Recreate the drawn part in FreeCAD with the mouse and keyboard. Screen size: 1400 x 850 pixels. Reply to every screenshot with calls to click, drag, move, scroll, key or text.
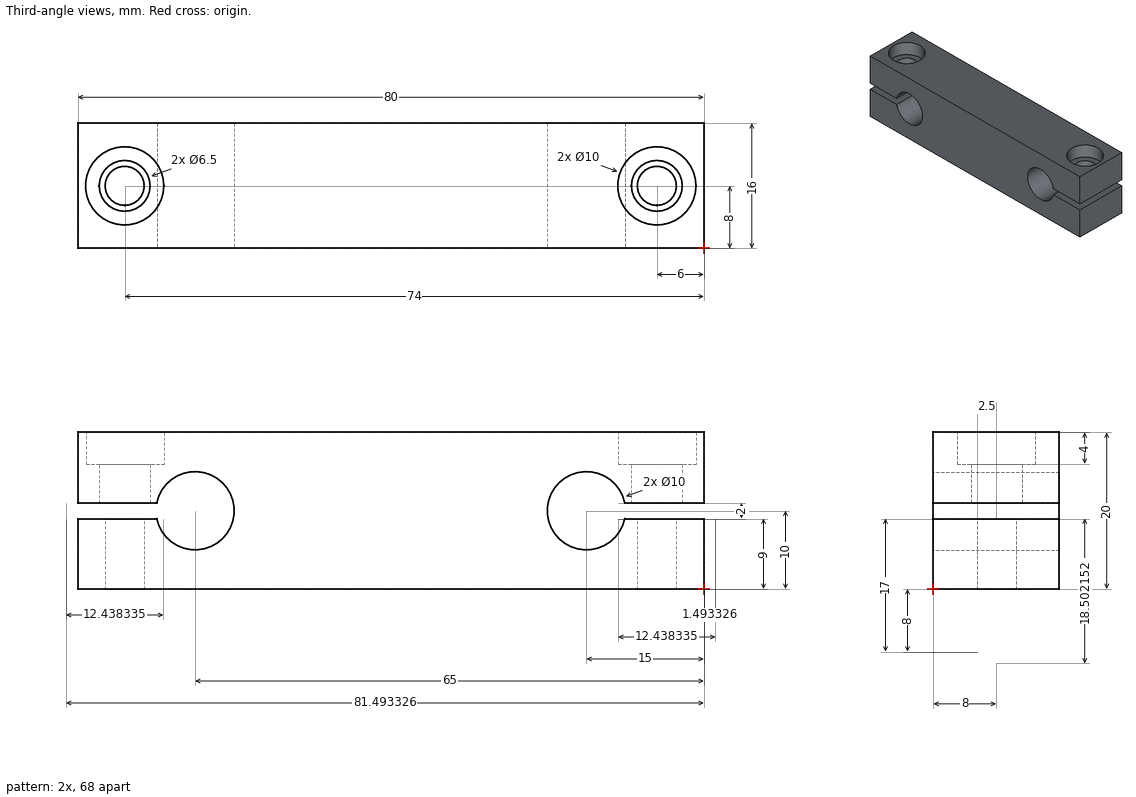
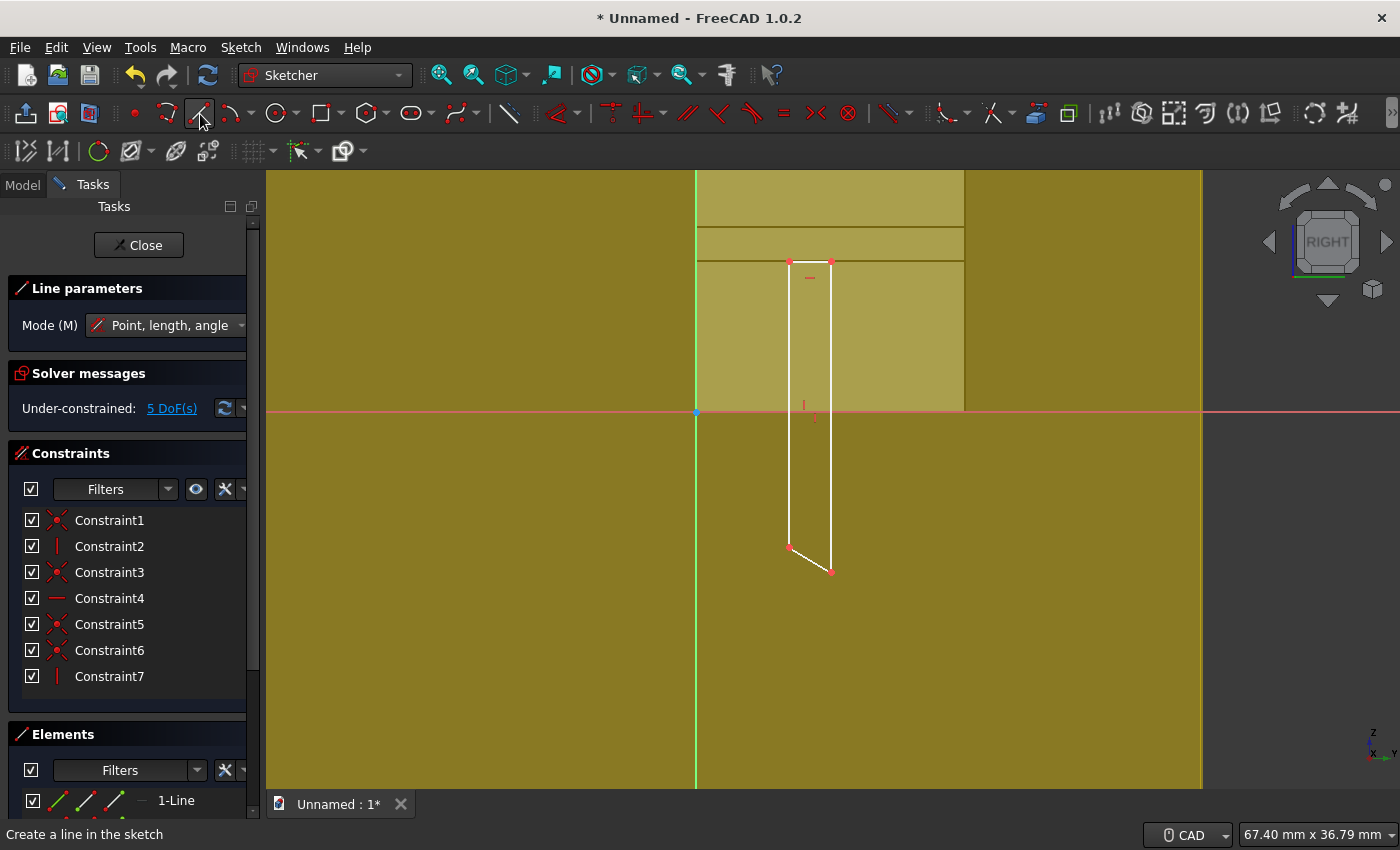
click(831, 603)
click(831, 697)
key(Escape)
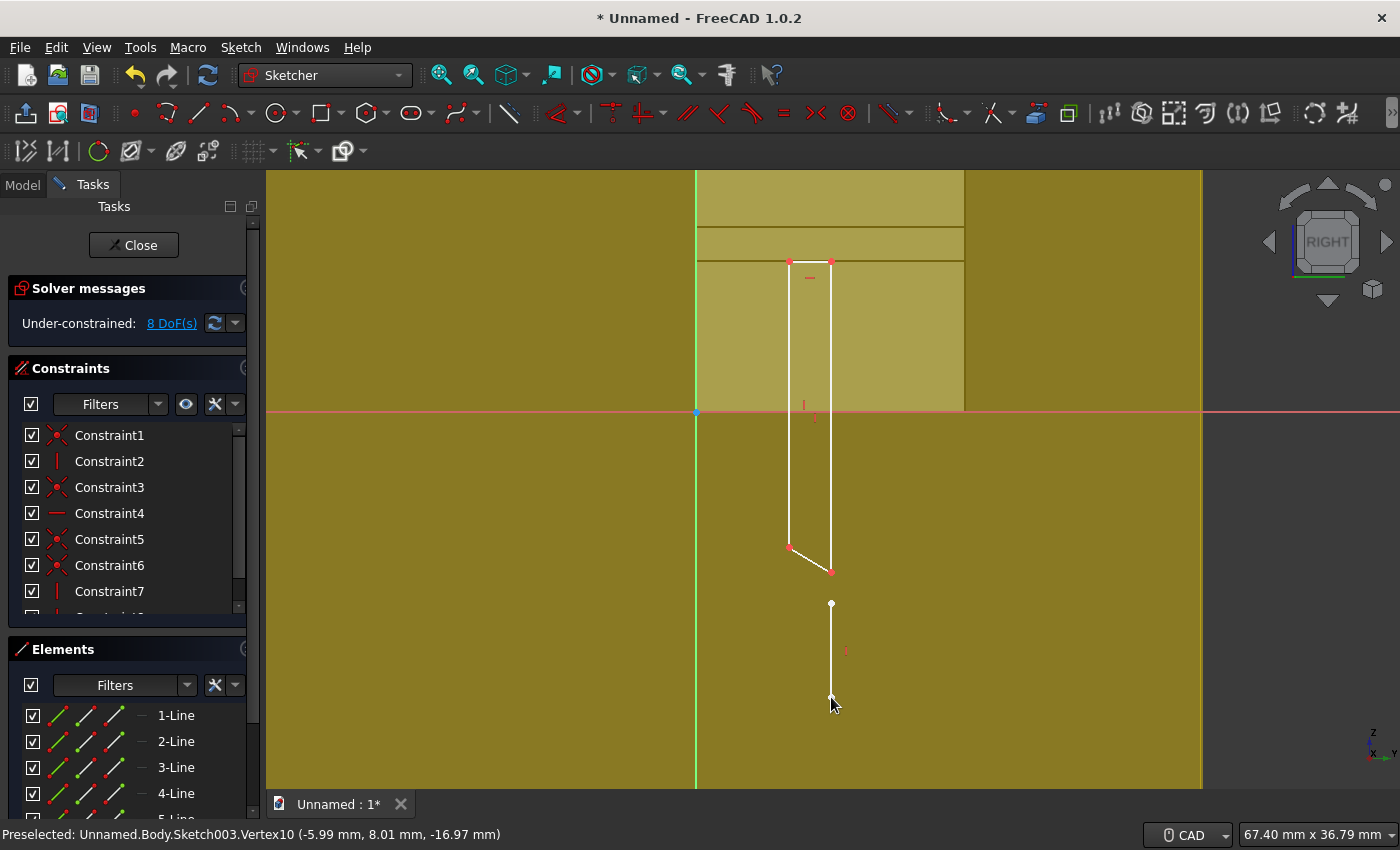
click(831, 632)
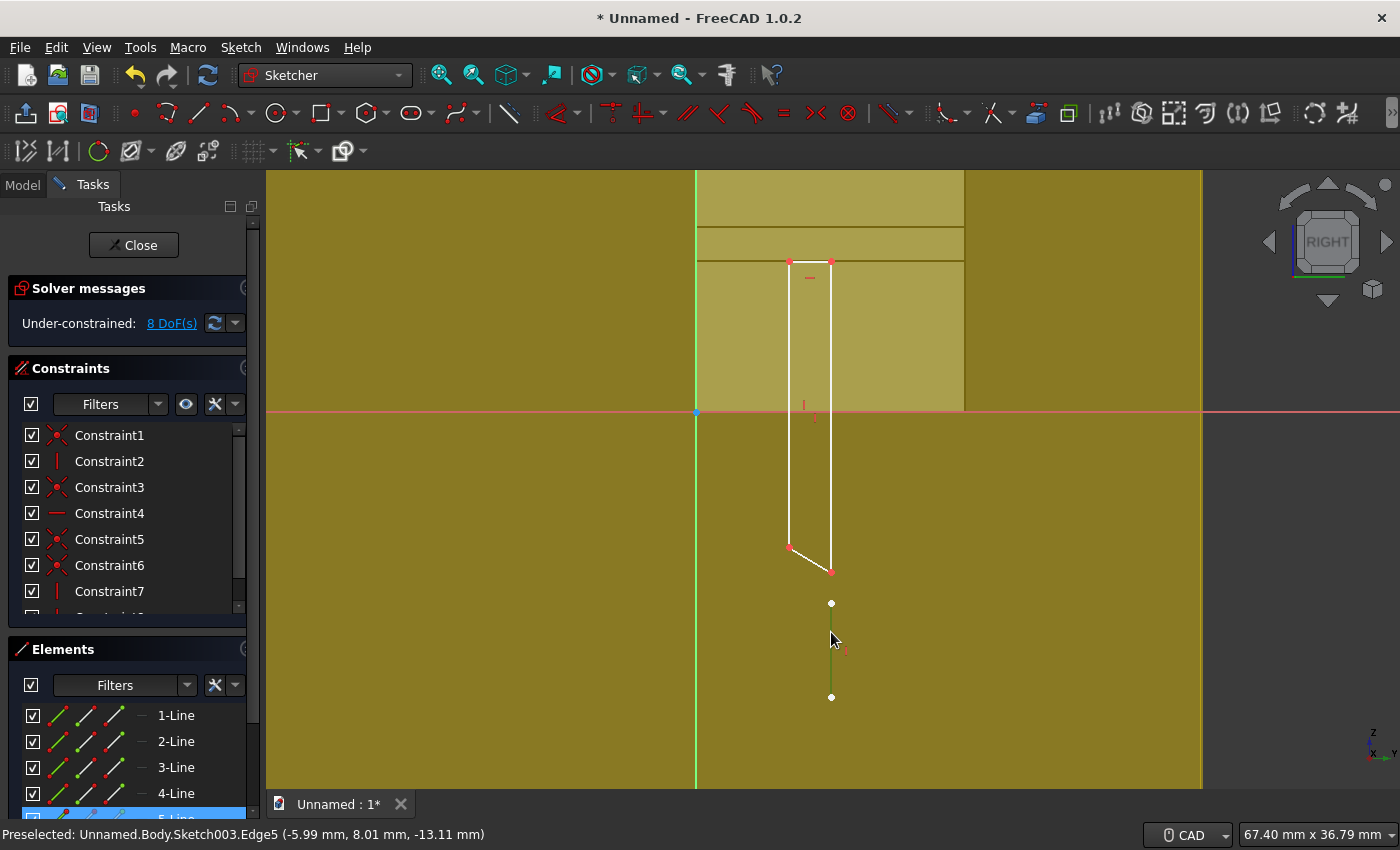
click(510, 114)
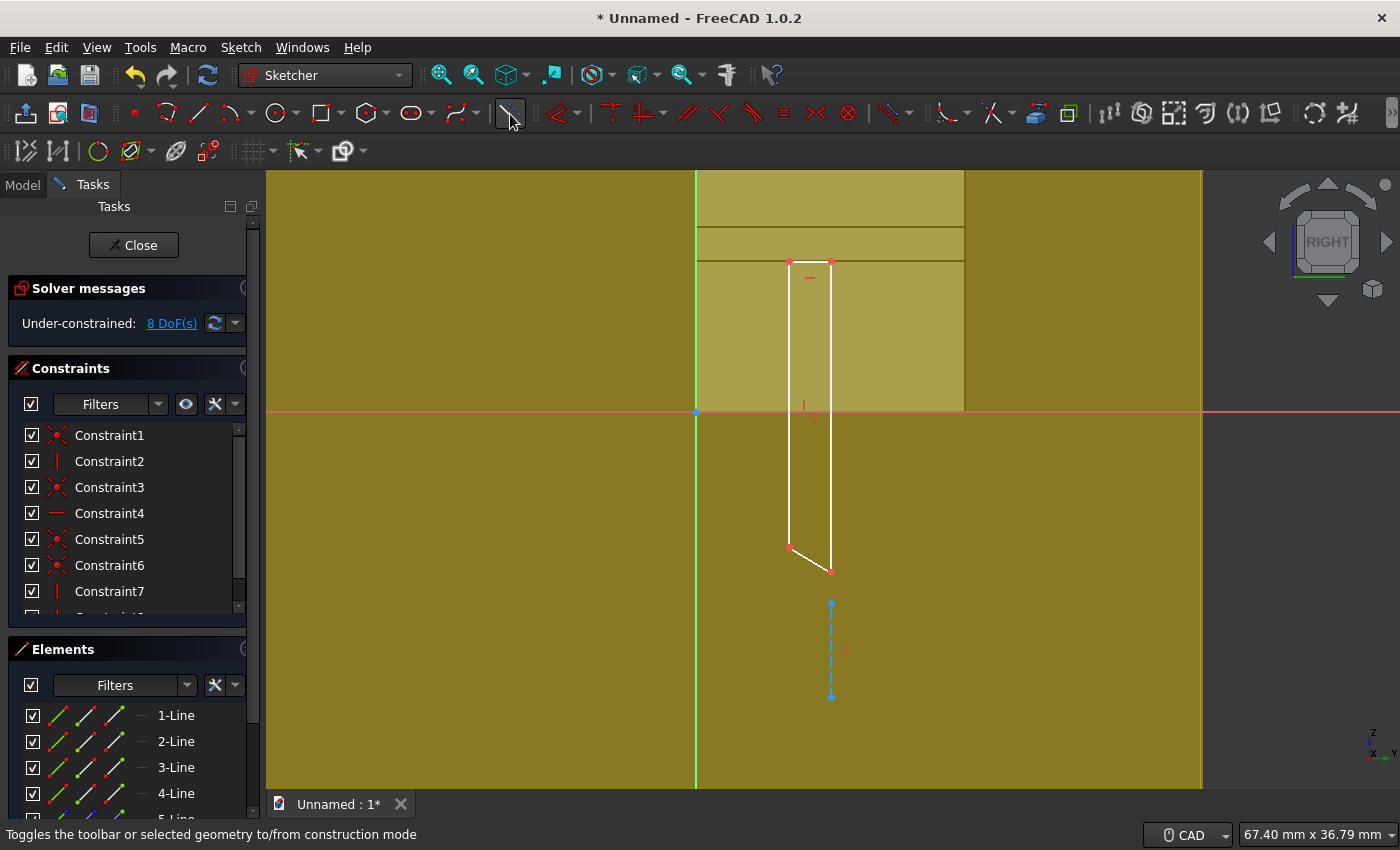
click(556, 114)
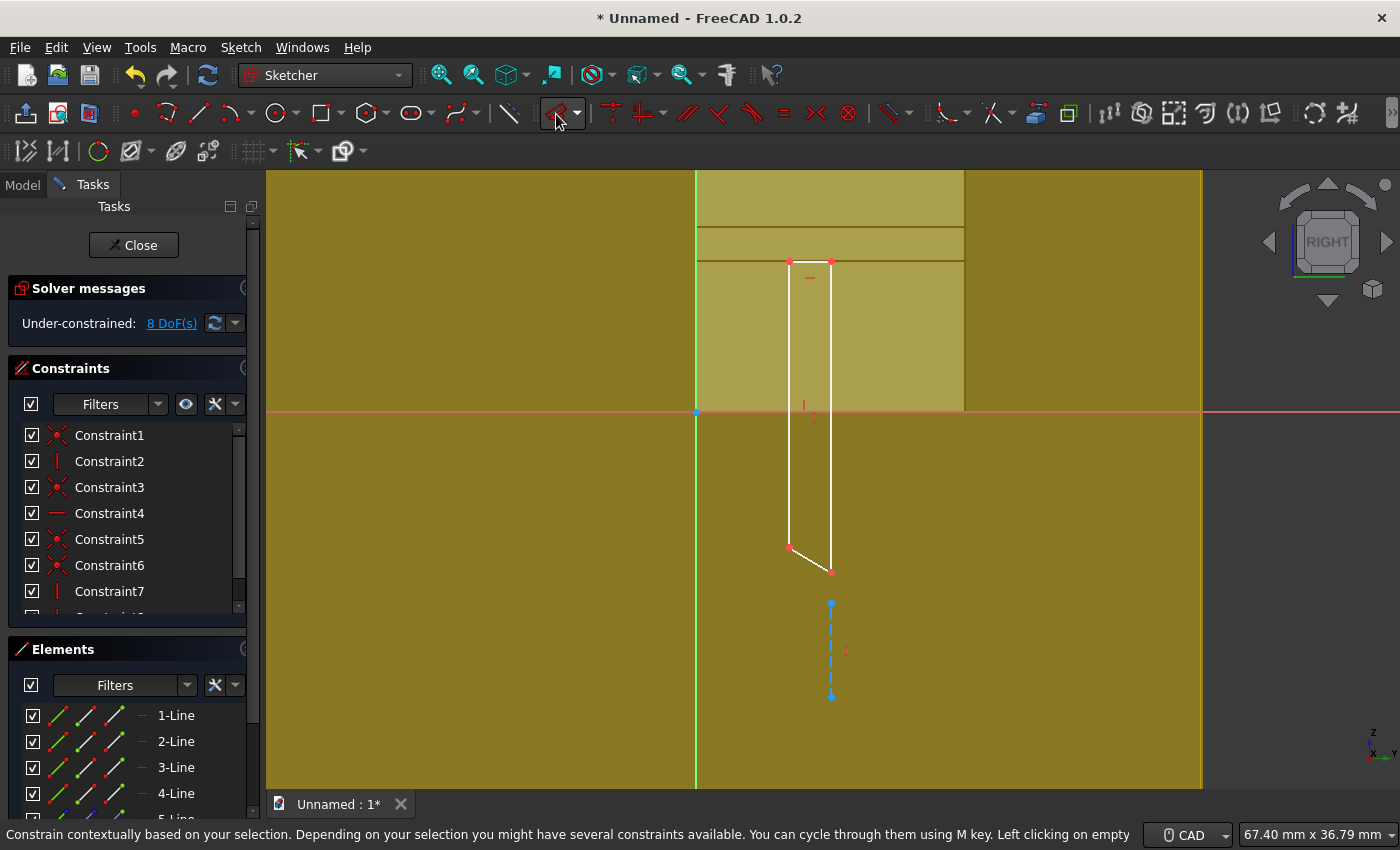
click(789, 348)
click(755, 339)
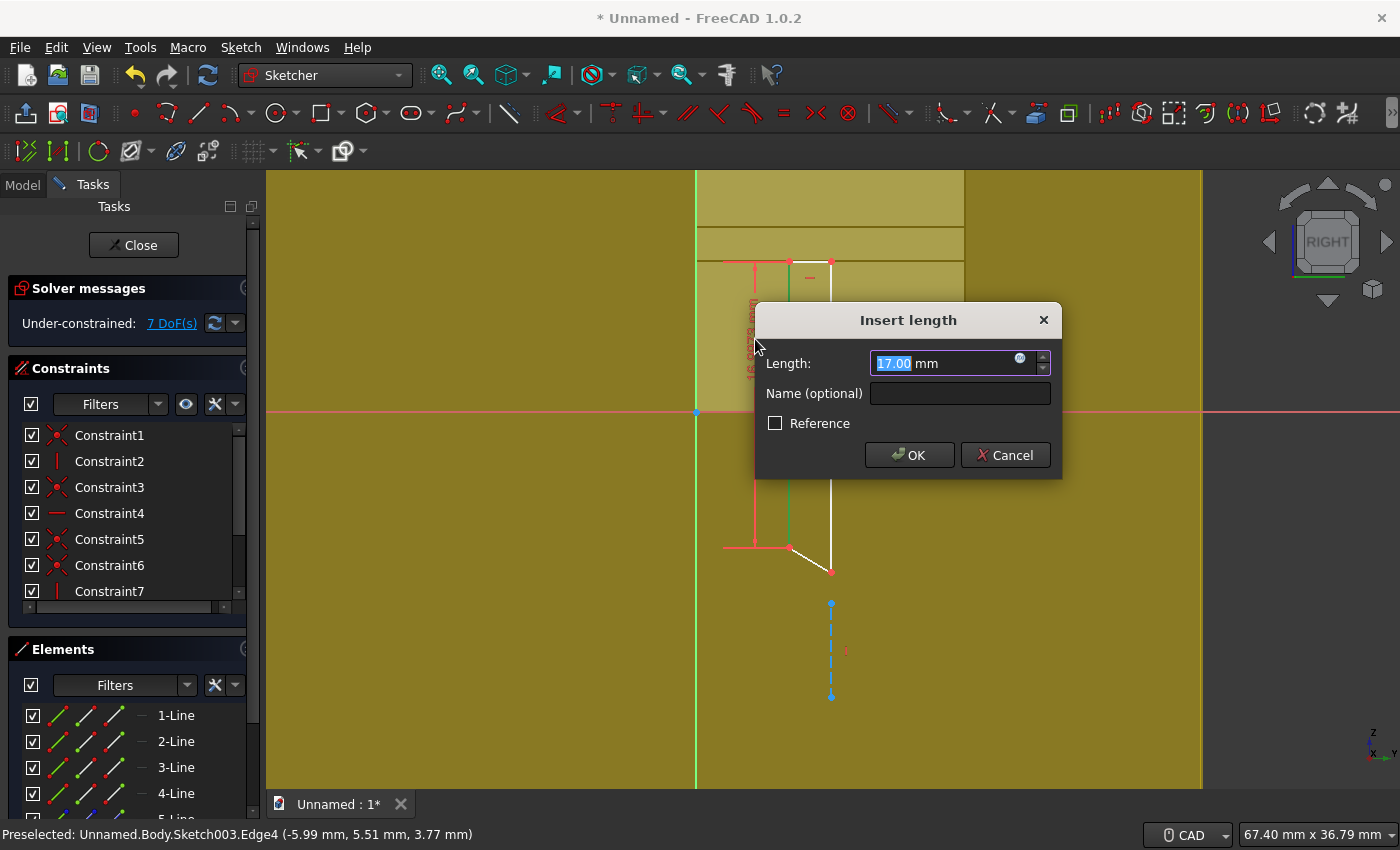
text(17)
key(Return)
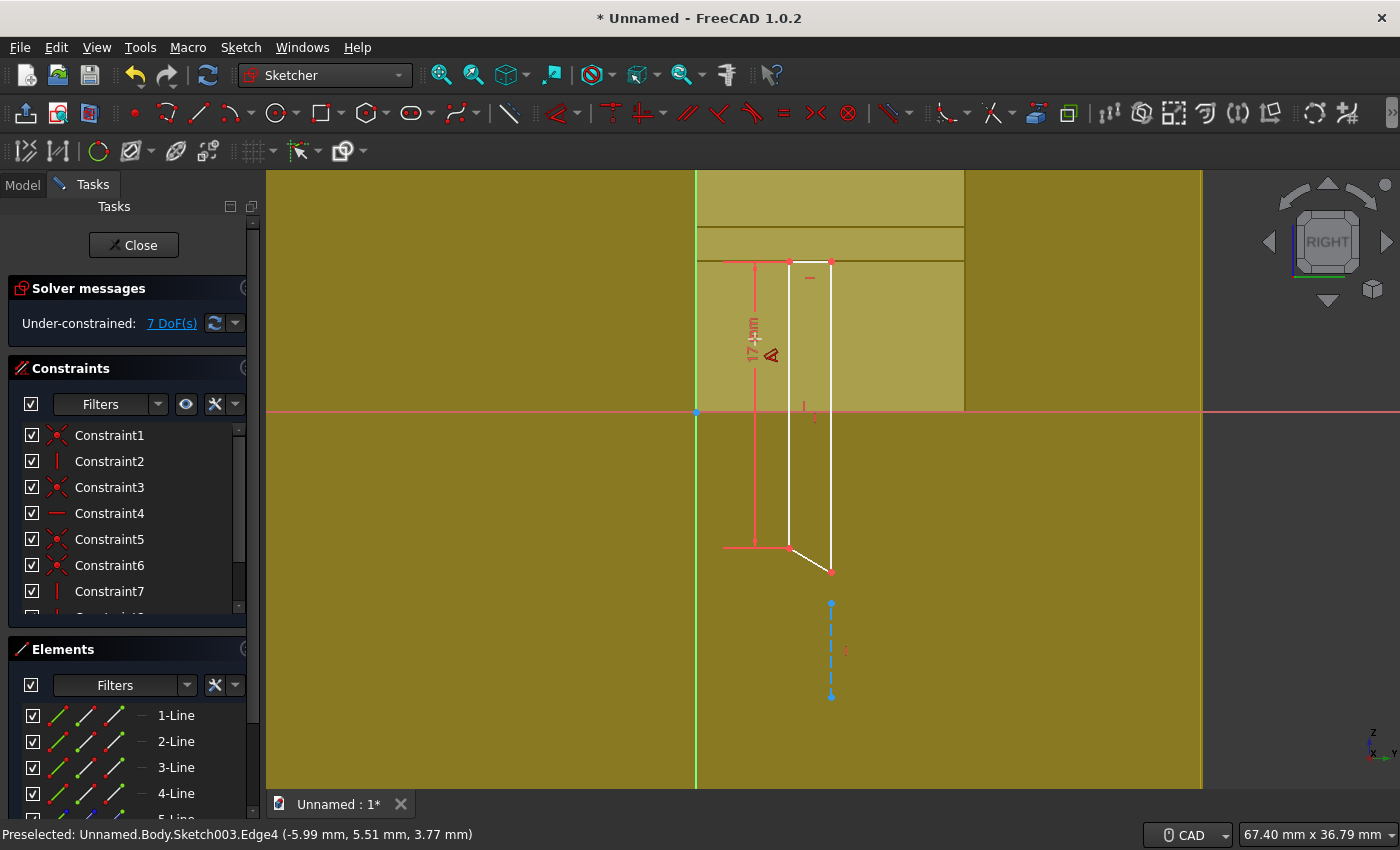
click(789, 548)
click(662, 480)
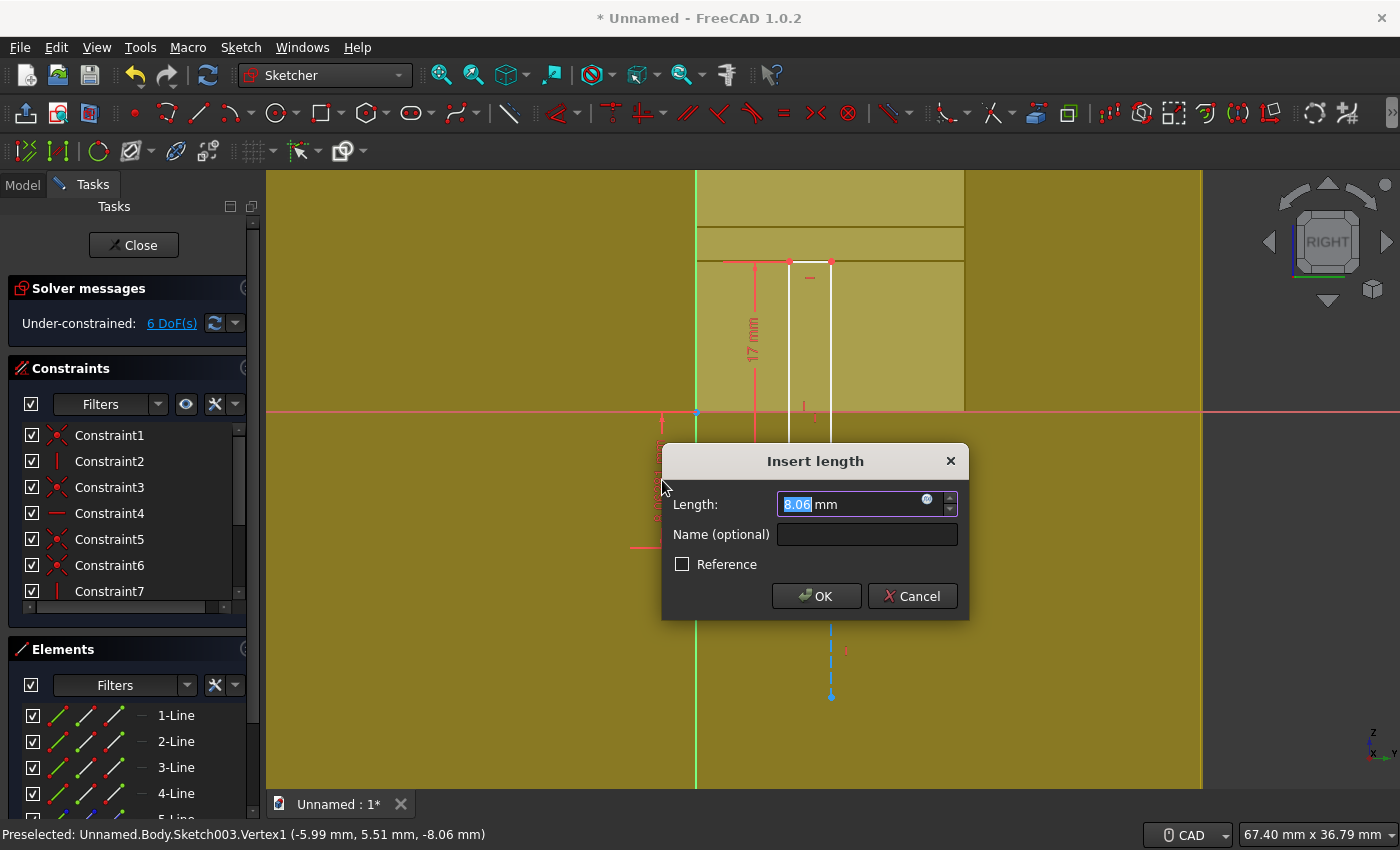
text(8)
key(Return)